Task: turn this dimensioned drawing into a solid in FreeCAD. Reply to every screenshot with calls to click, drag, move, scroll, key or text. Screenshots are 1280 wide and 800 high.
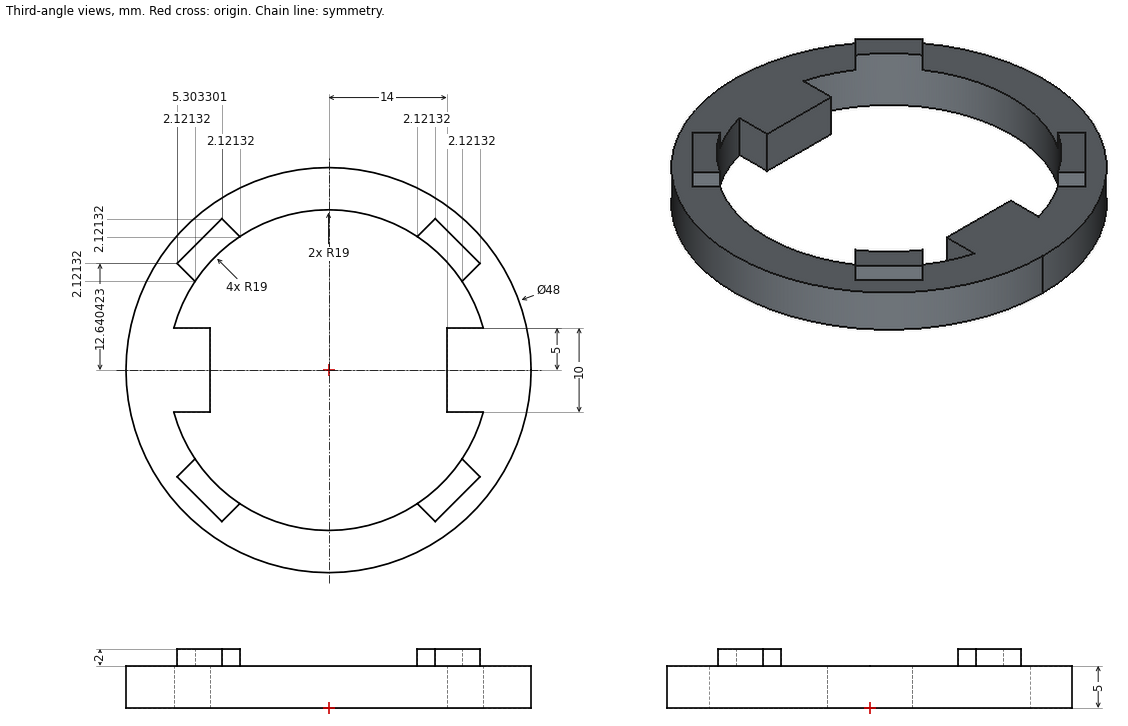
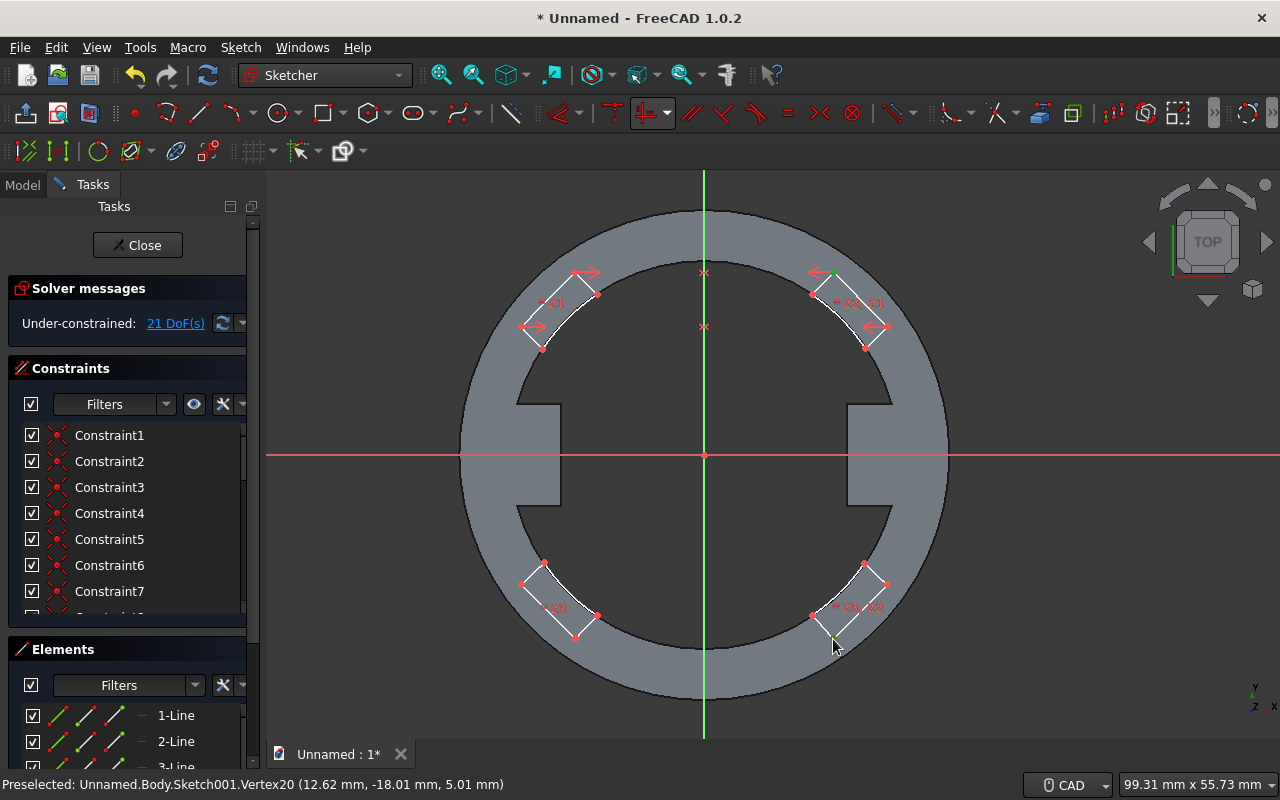
click(353, 455)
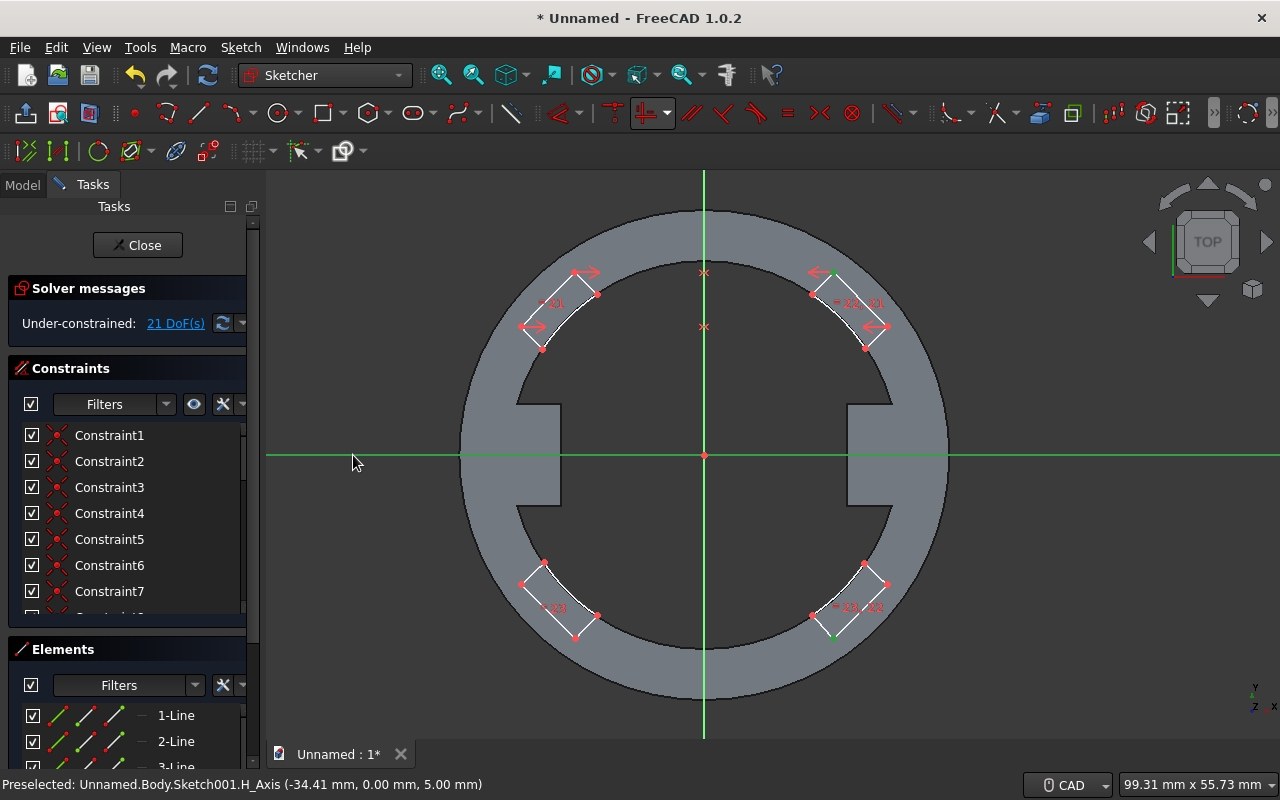
key(s)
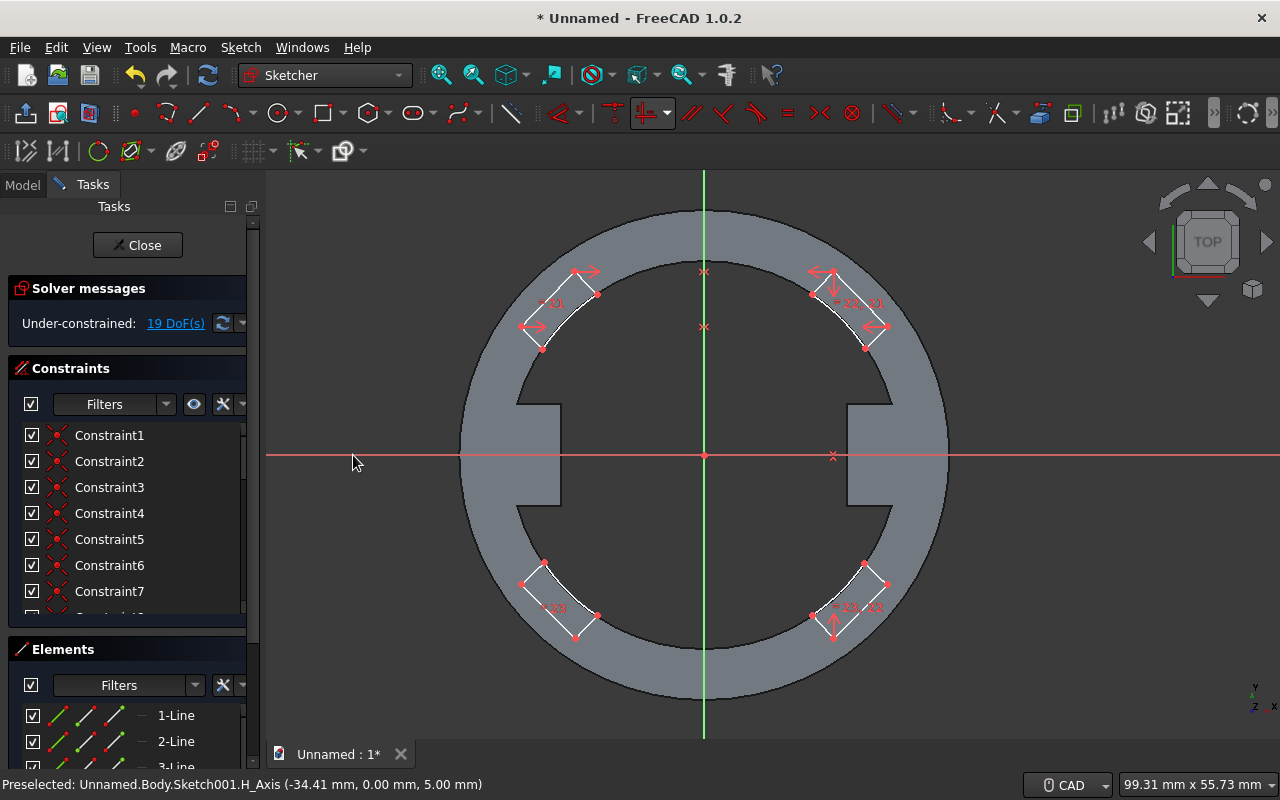
click(888, 327)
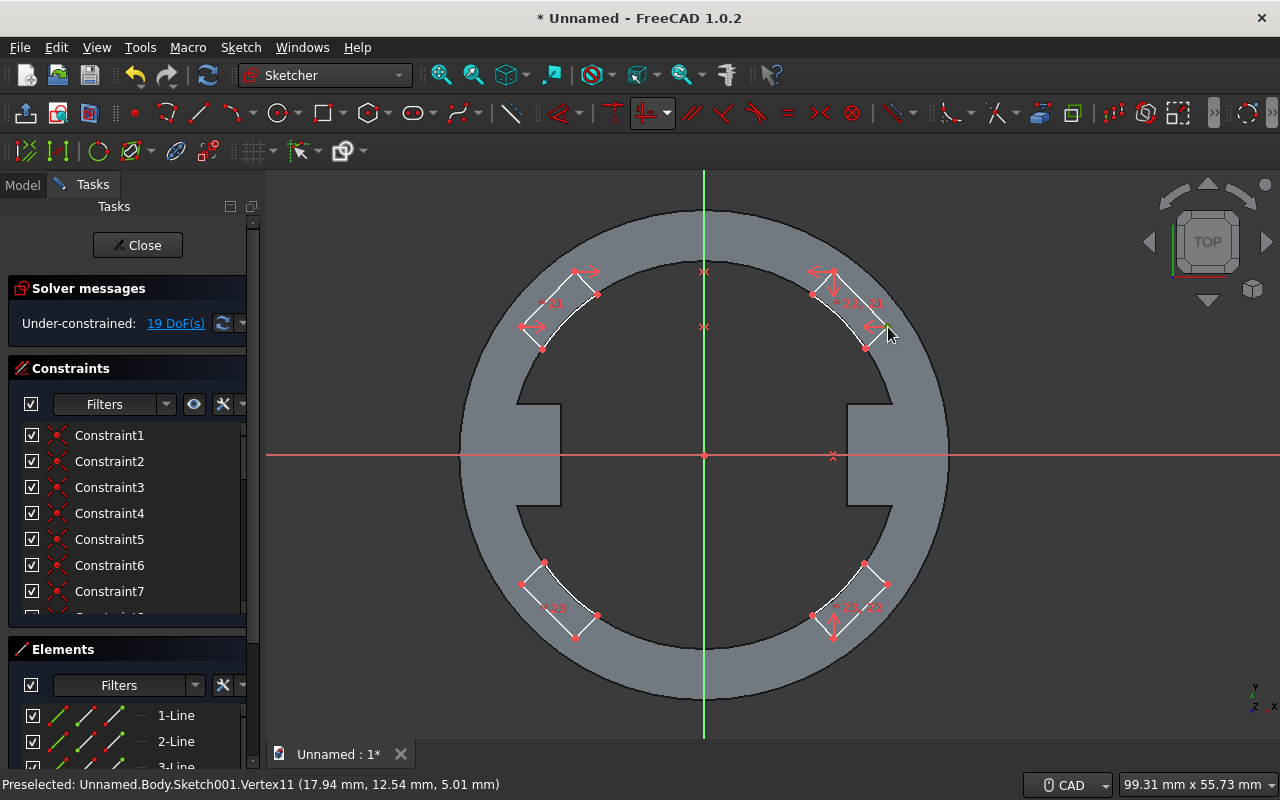
click(887, 585)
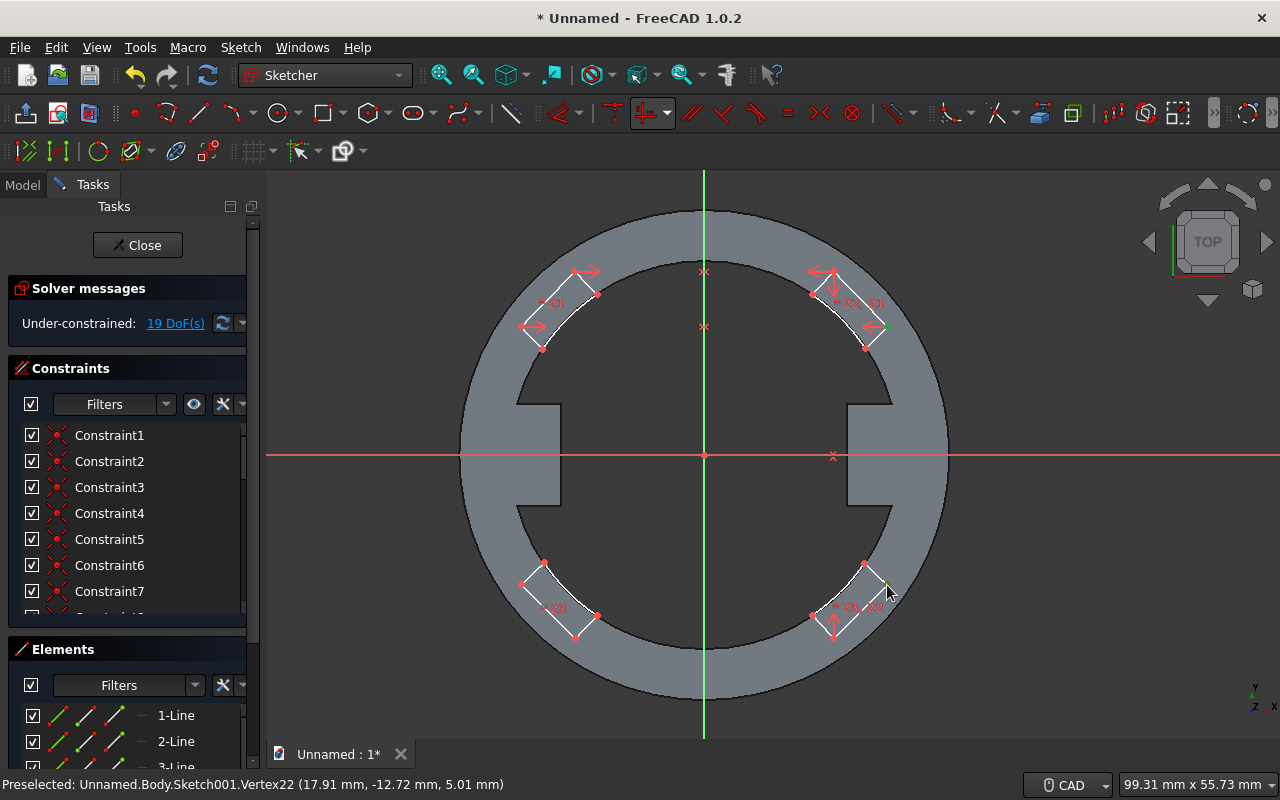
click(353, 455)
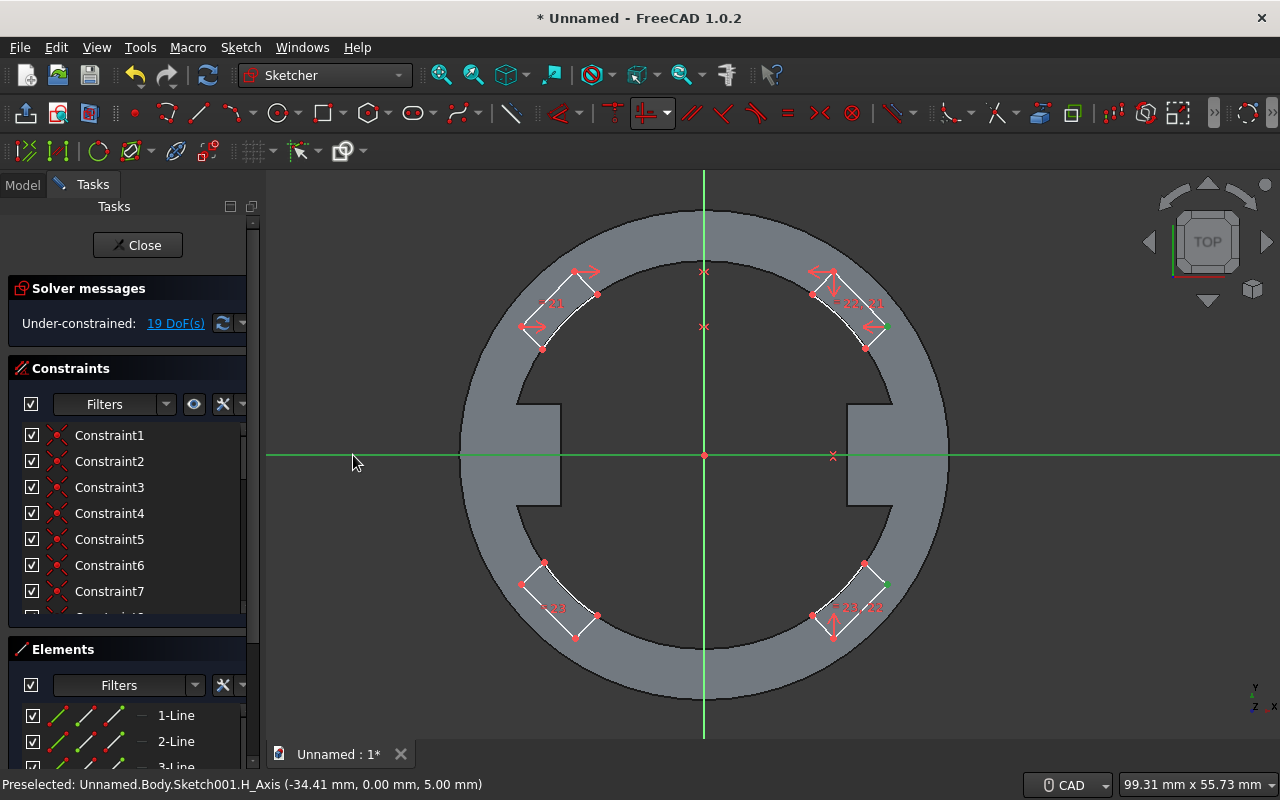
click(820, 114)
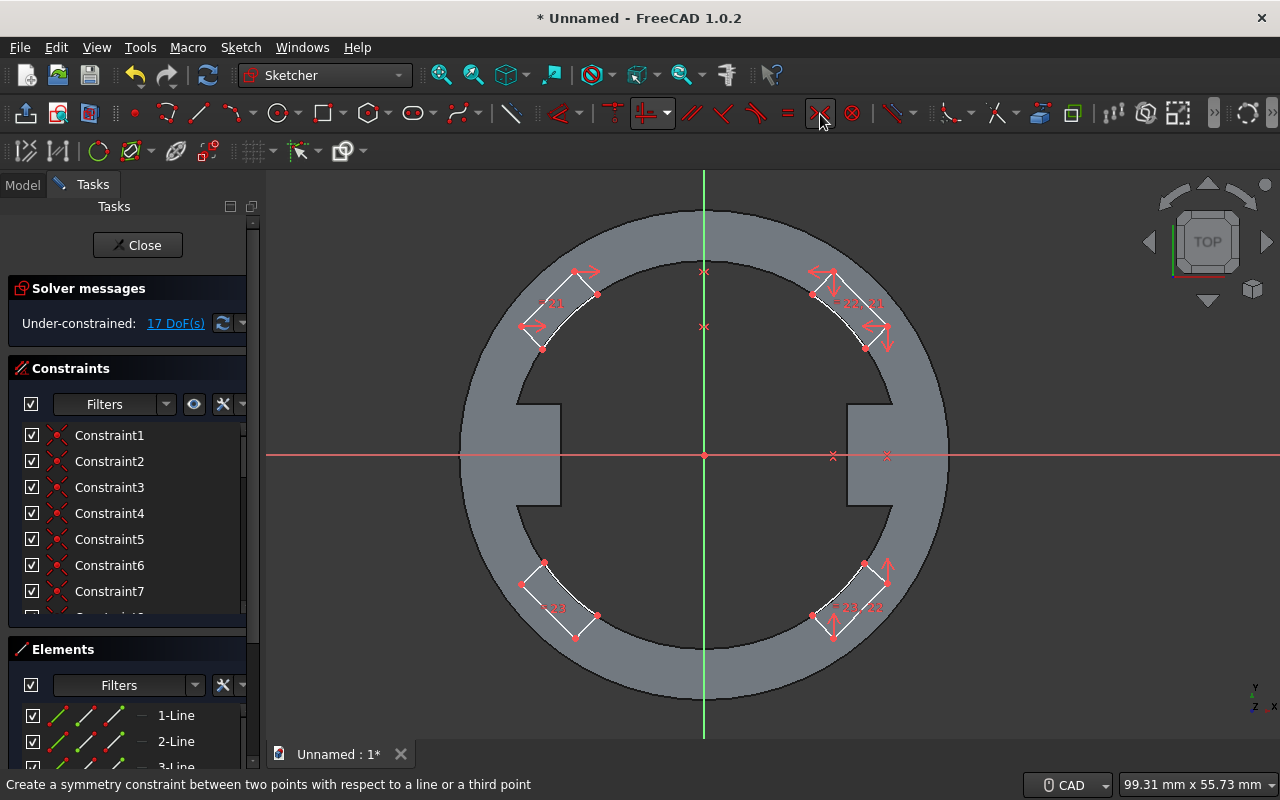
click(521, 326)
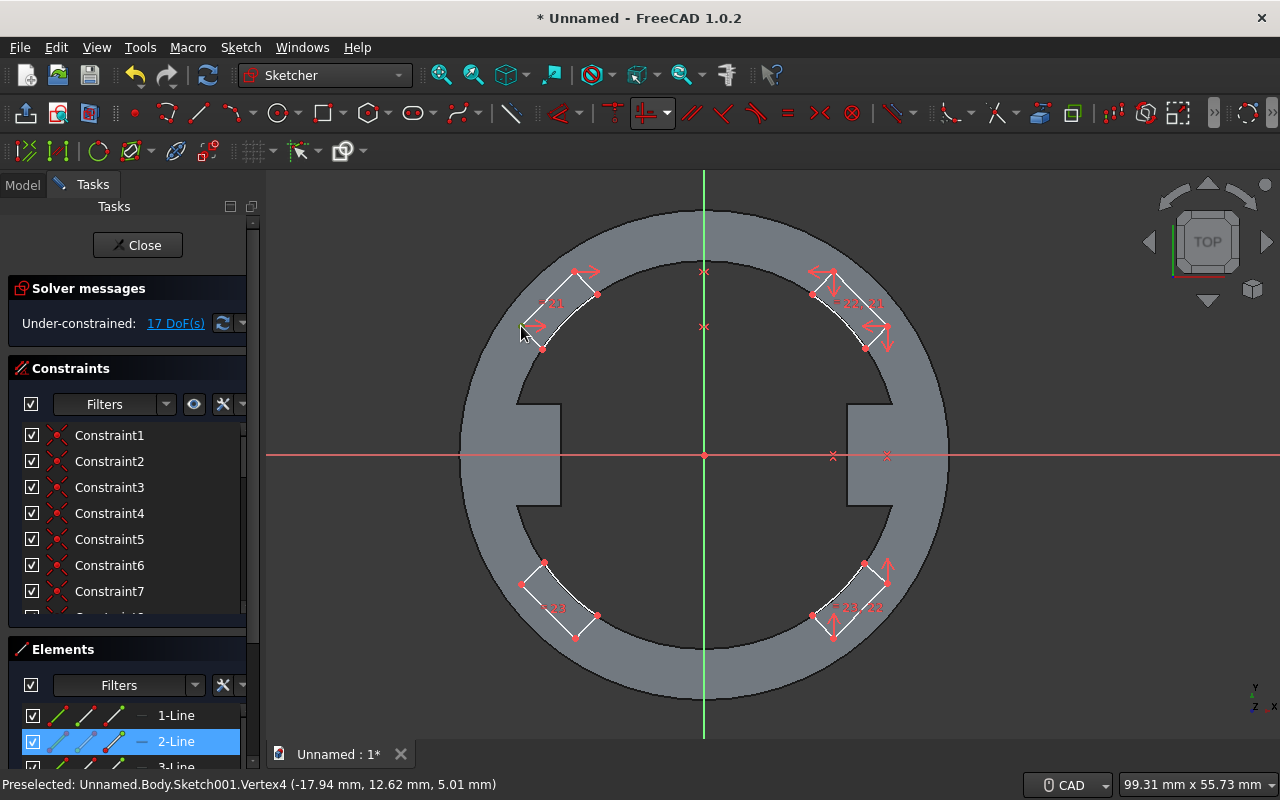
click(521, 585)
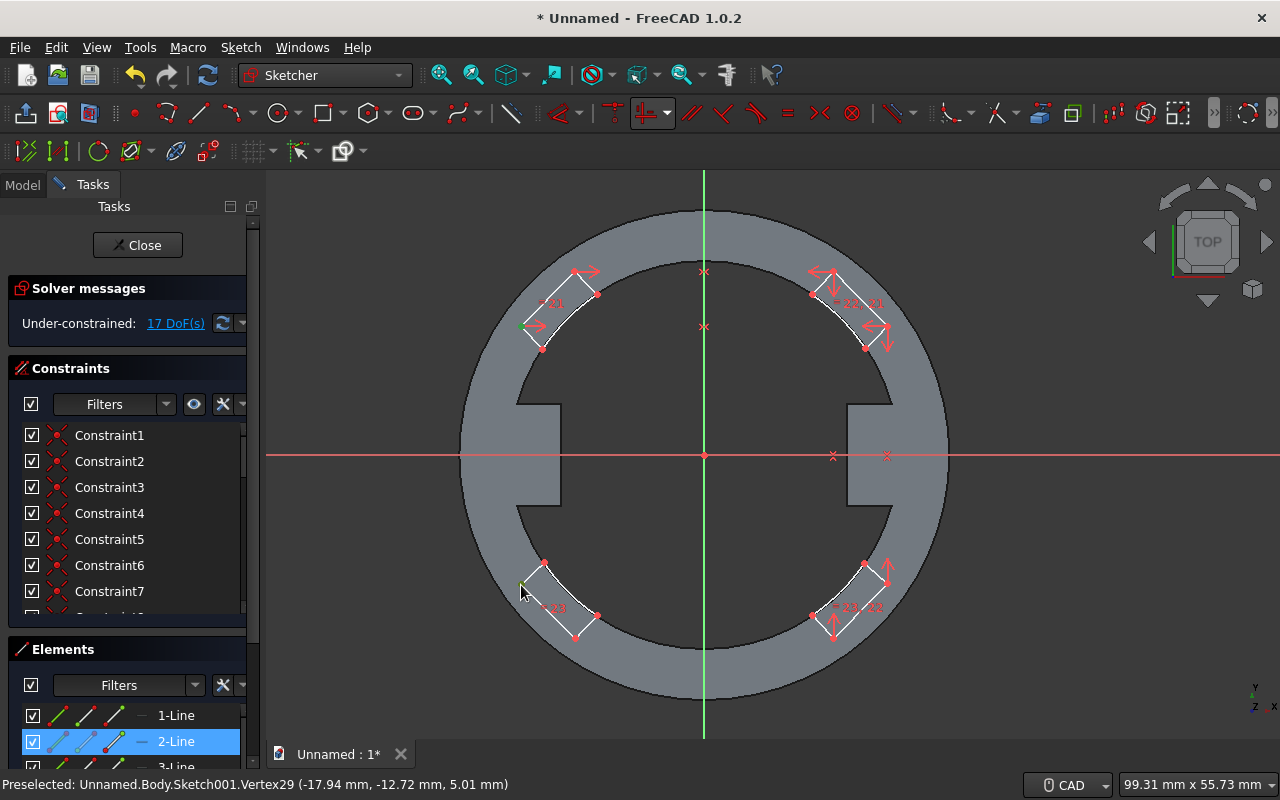
click(353, 455)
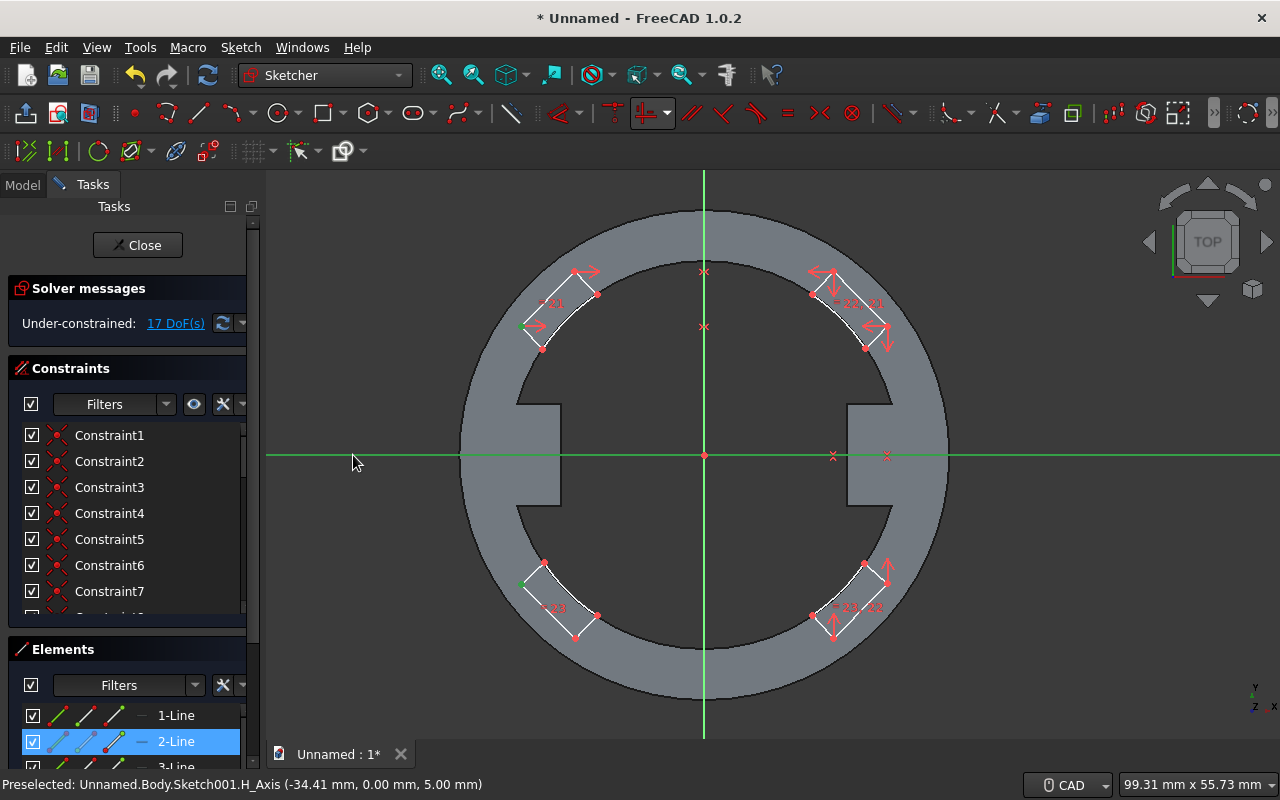
key(s)